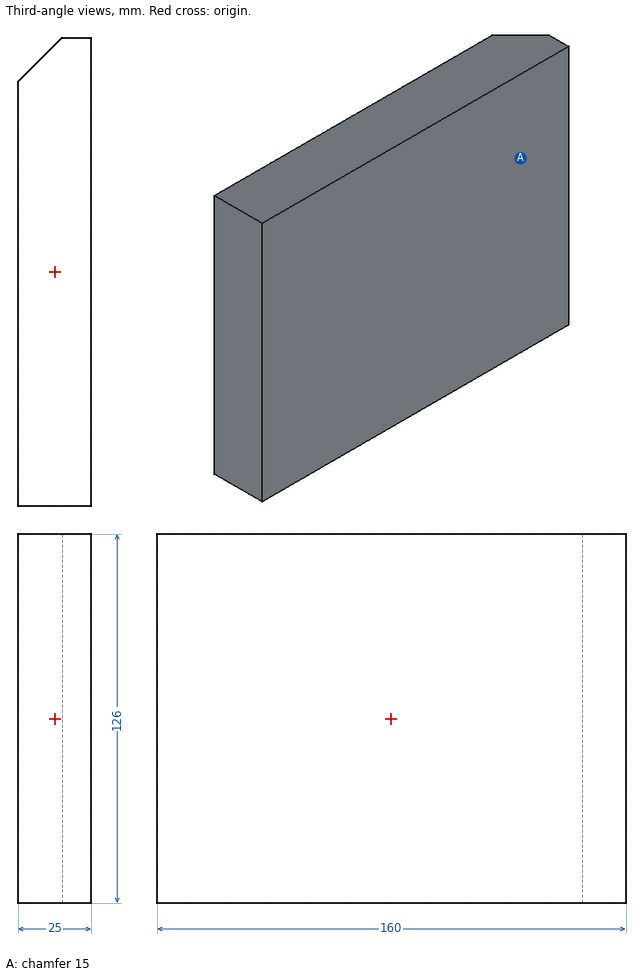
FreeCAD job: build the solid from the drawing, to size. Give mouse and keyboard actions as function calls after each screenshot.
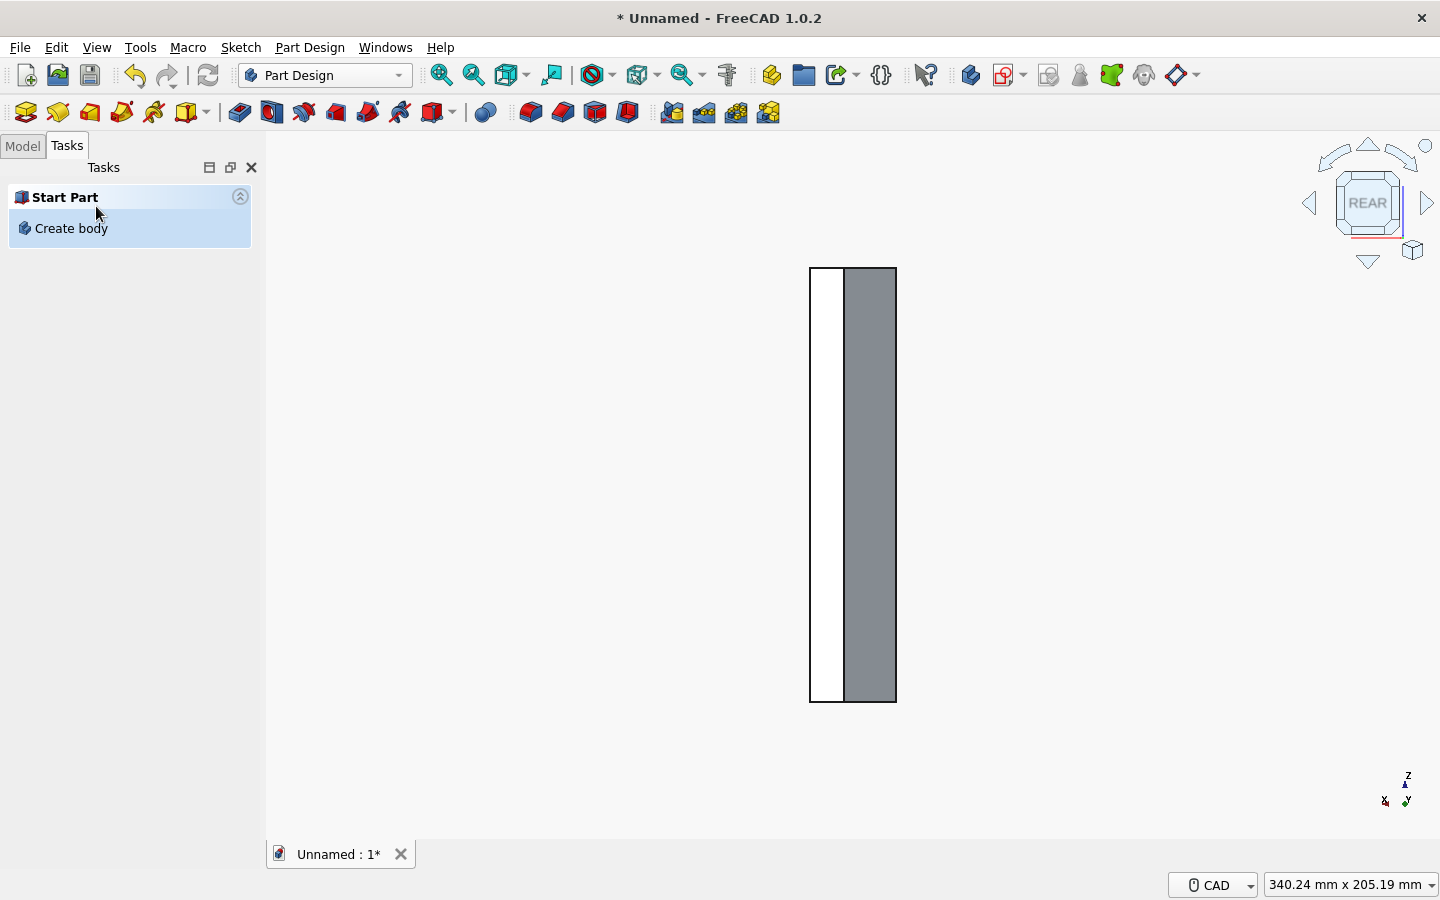
key(0)